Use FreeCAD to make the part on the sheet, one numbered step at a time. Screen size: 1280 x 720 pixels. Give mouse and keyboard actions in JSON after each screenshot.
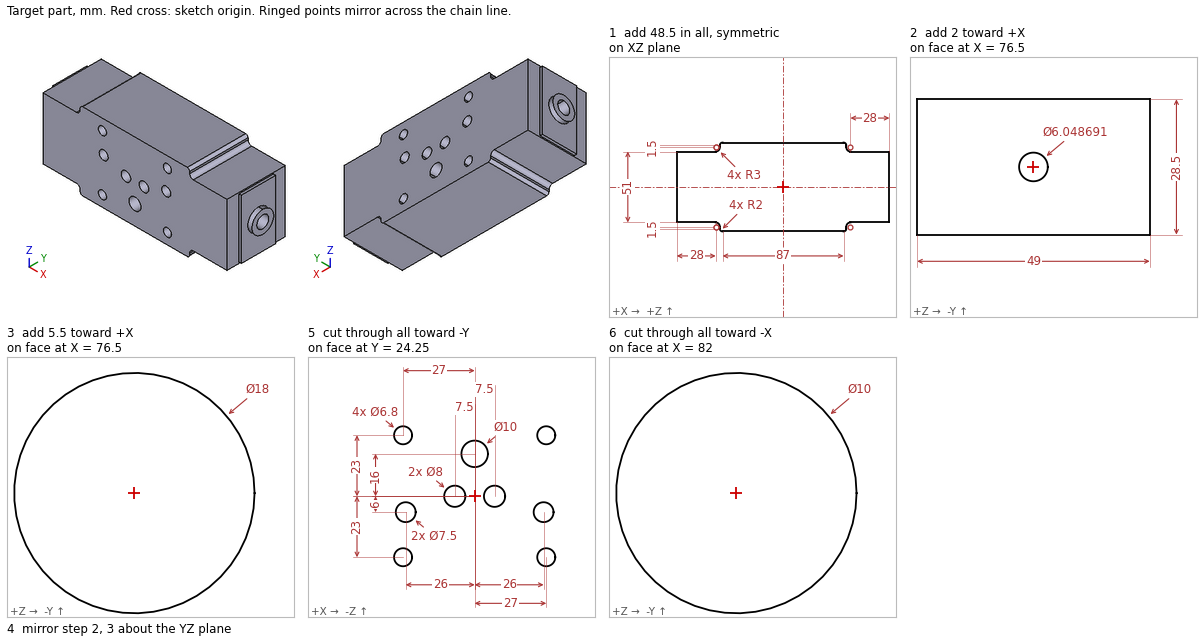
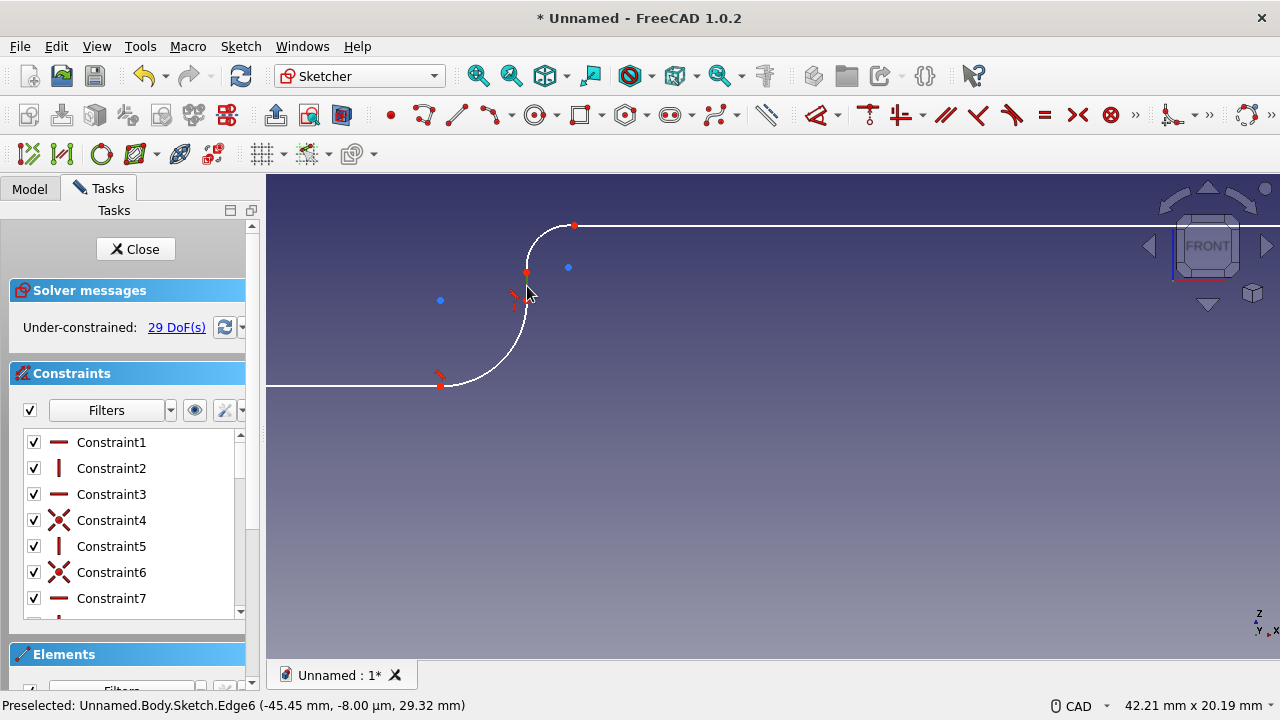
{"action": "left_click", "coordinate": [552, 229]}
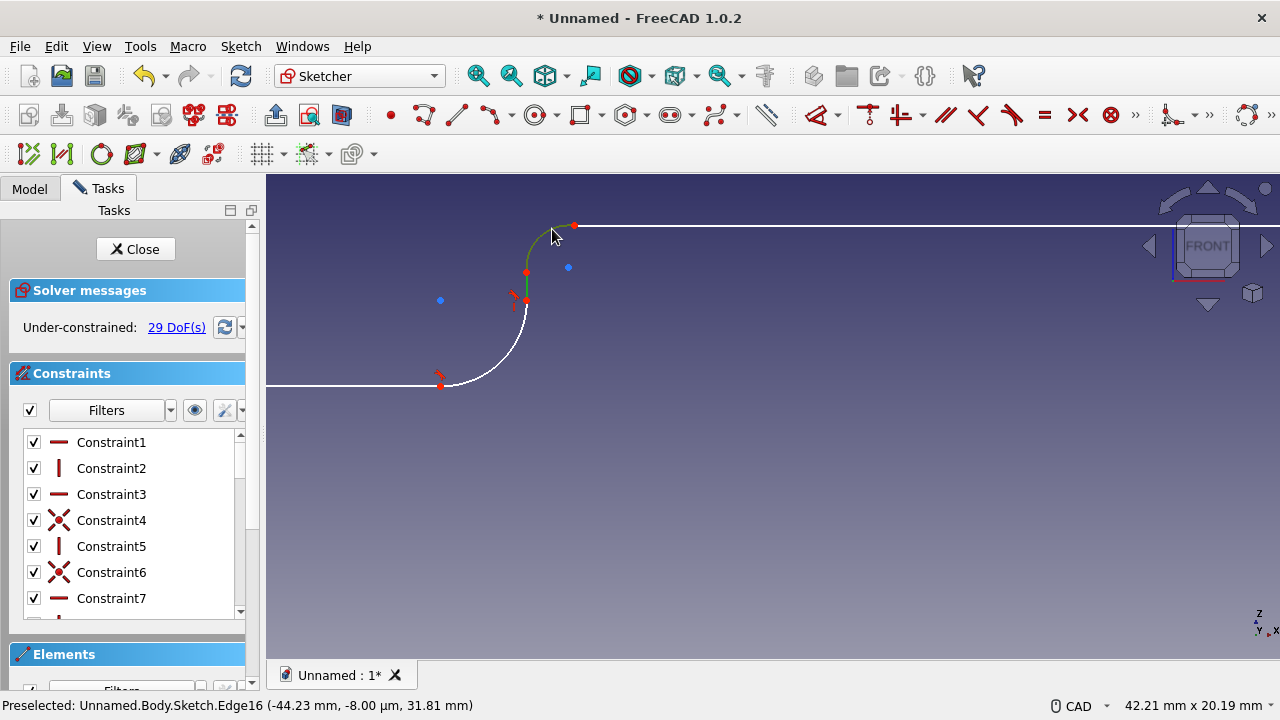
{"action": "left_click", "coordinate": [1012, 116]}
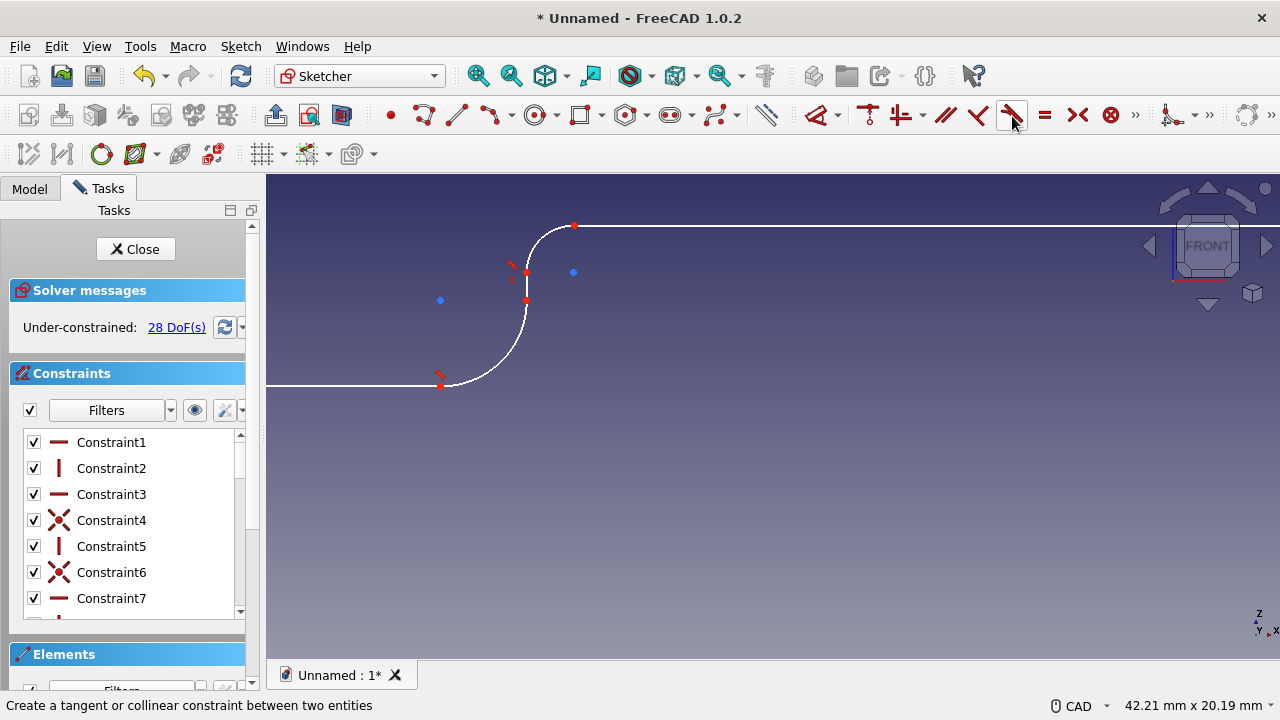
{"action": "scroll", "coordinate": [523, 303], "scroll_direction": "down", "scroll_amount": 9}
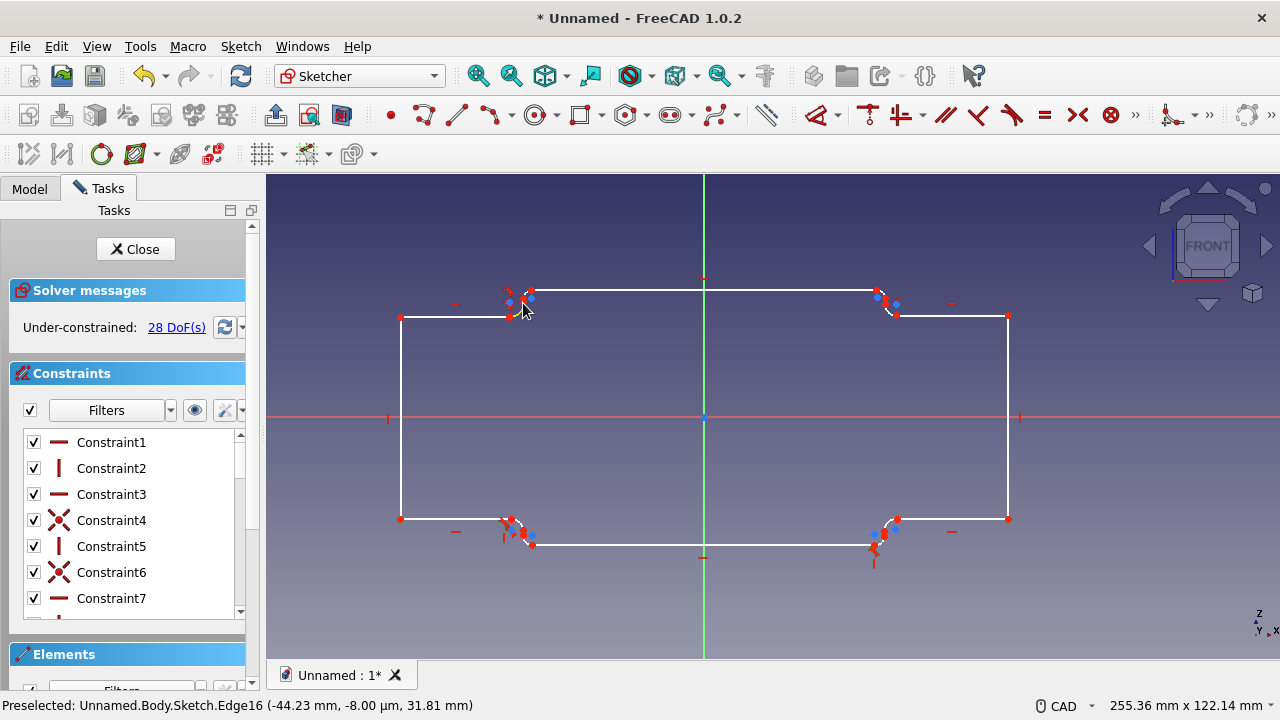
{"action": "left_click", "coordinate": [601, 290]}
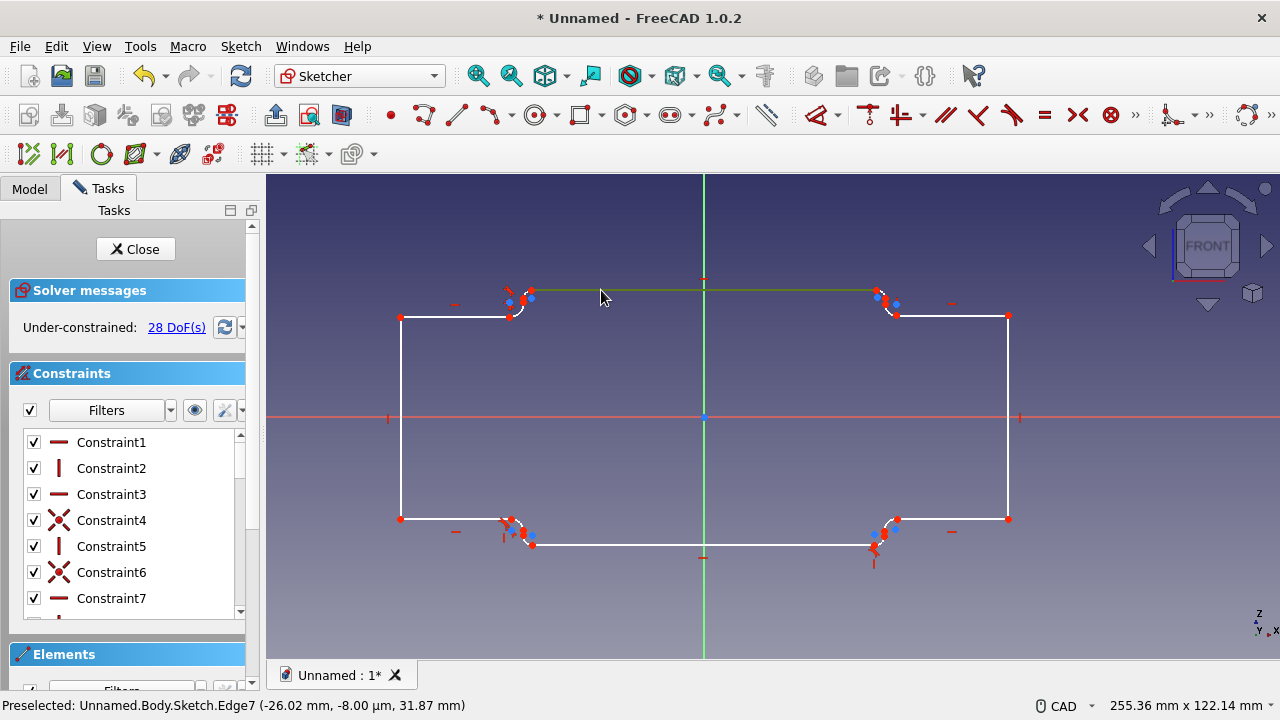
{"action": "scroll", "coordinate": [526, 293], "scroll_direction": "up", "scroll_amount": 5}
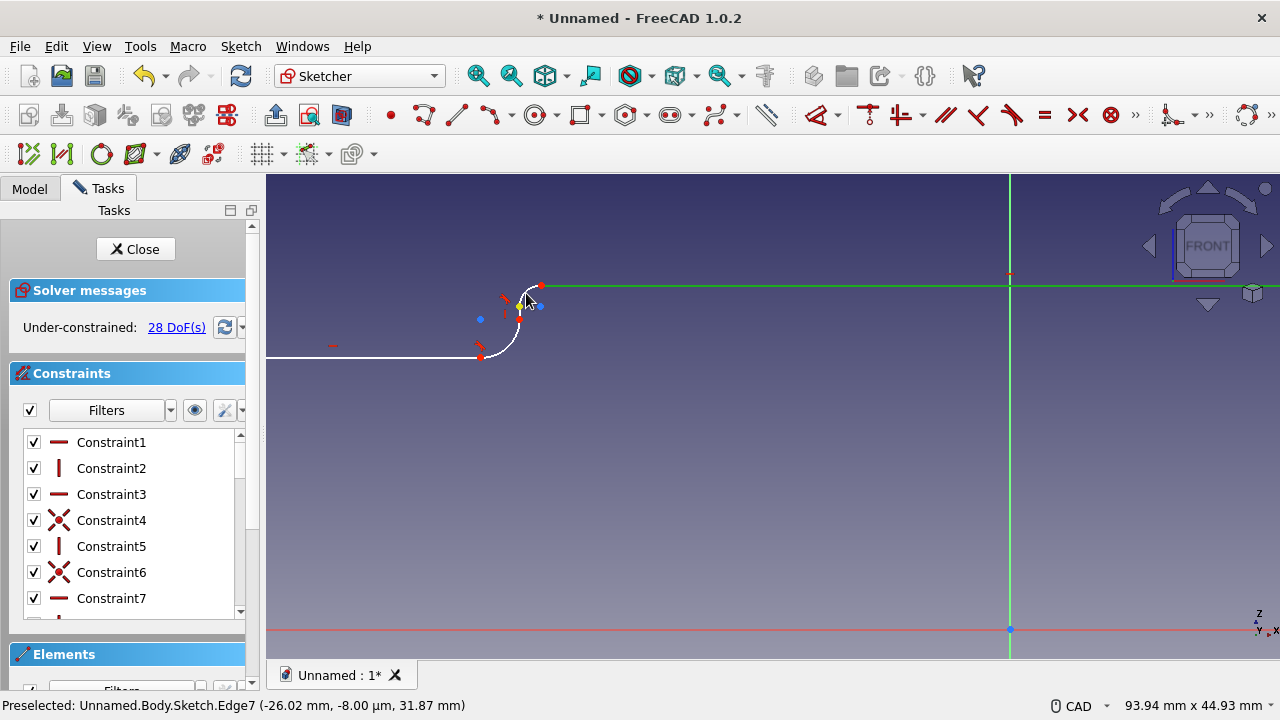
{"action": "left_click", "coordinate": [526, 292]}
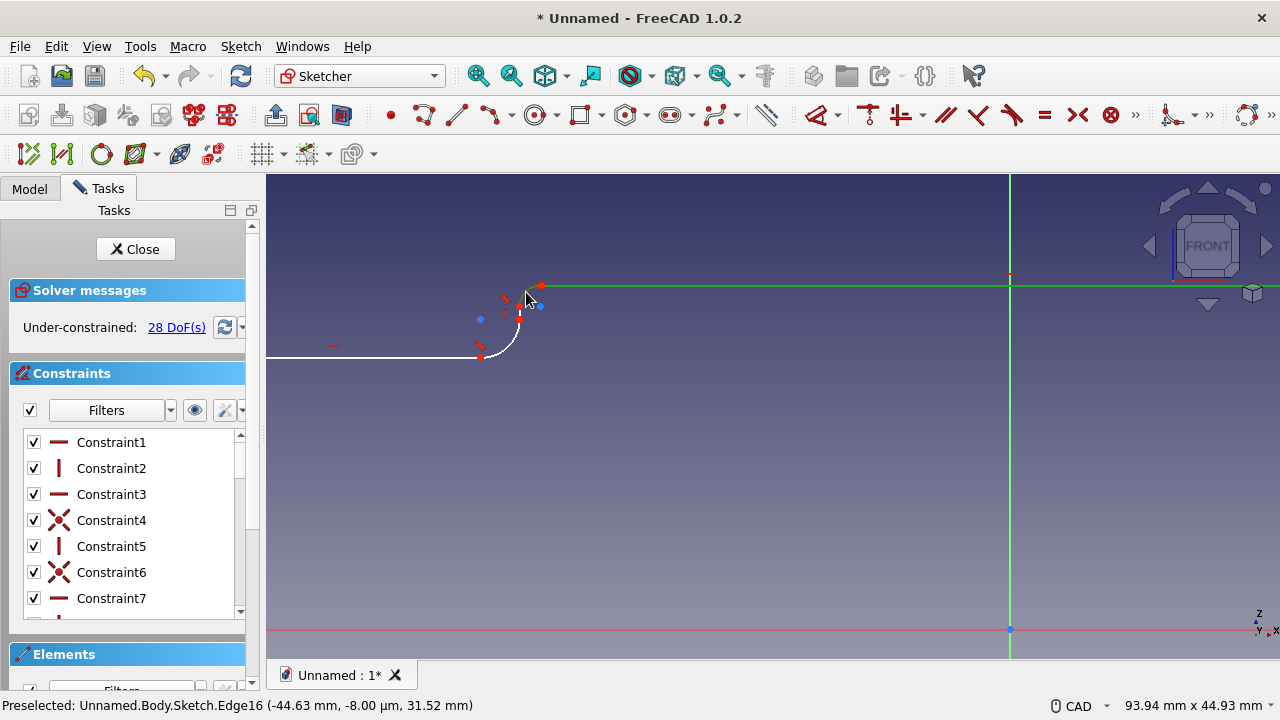
{"action": "left_click", "coordinate": [1012, 116]}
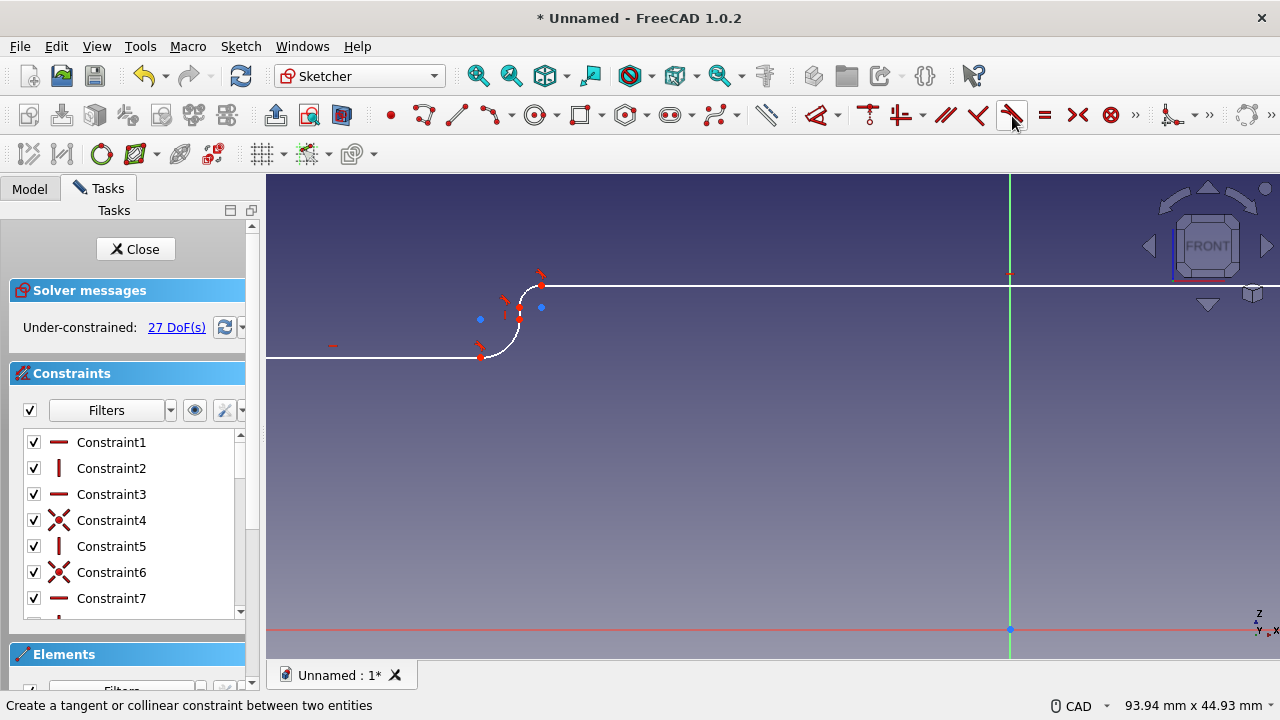
{"action": "left_click", "coordinate": [823, 286]}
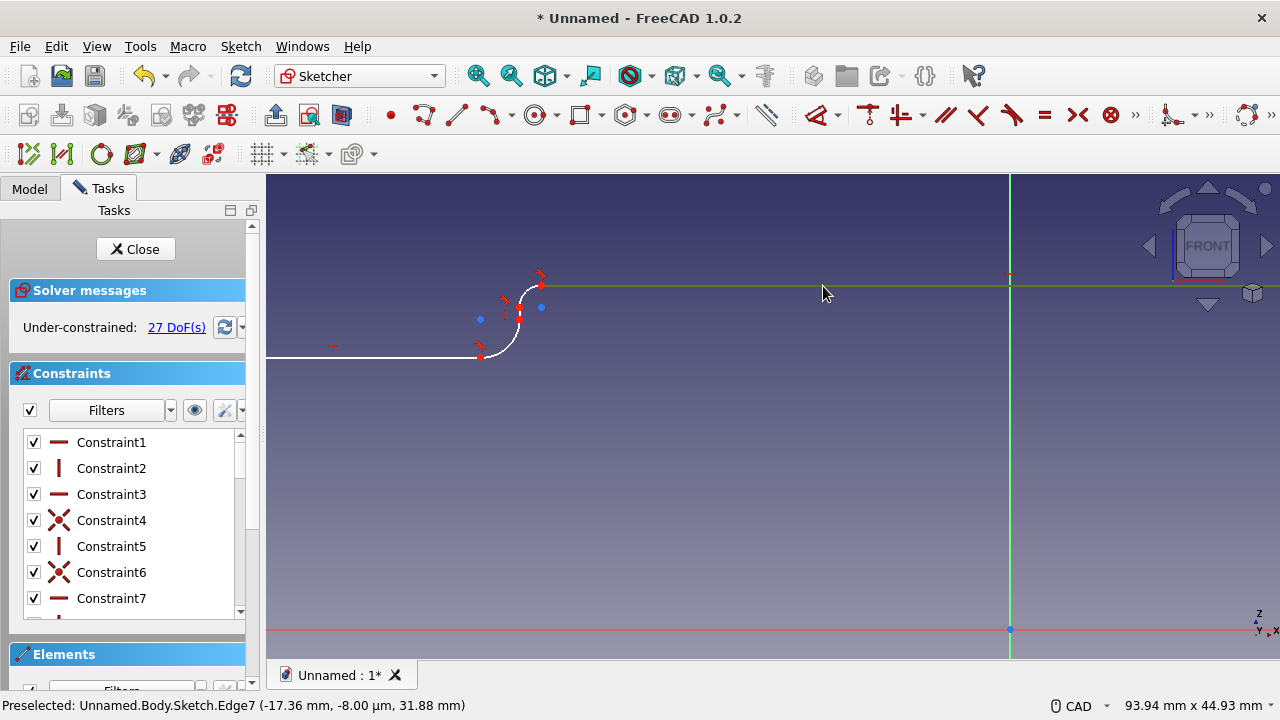
{"action": "scroll", "coordinate": [527, 292], "scroll_direction": "down", "scroll_amount": 5}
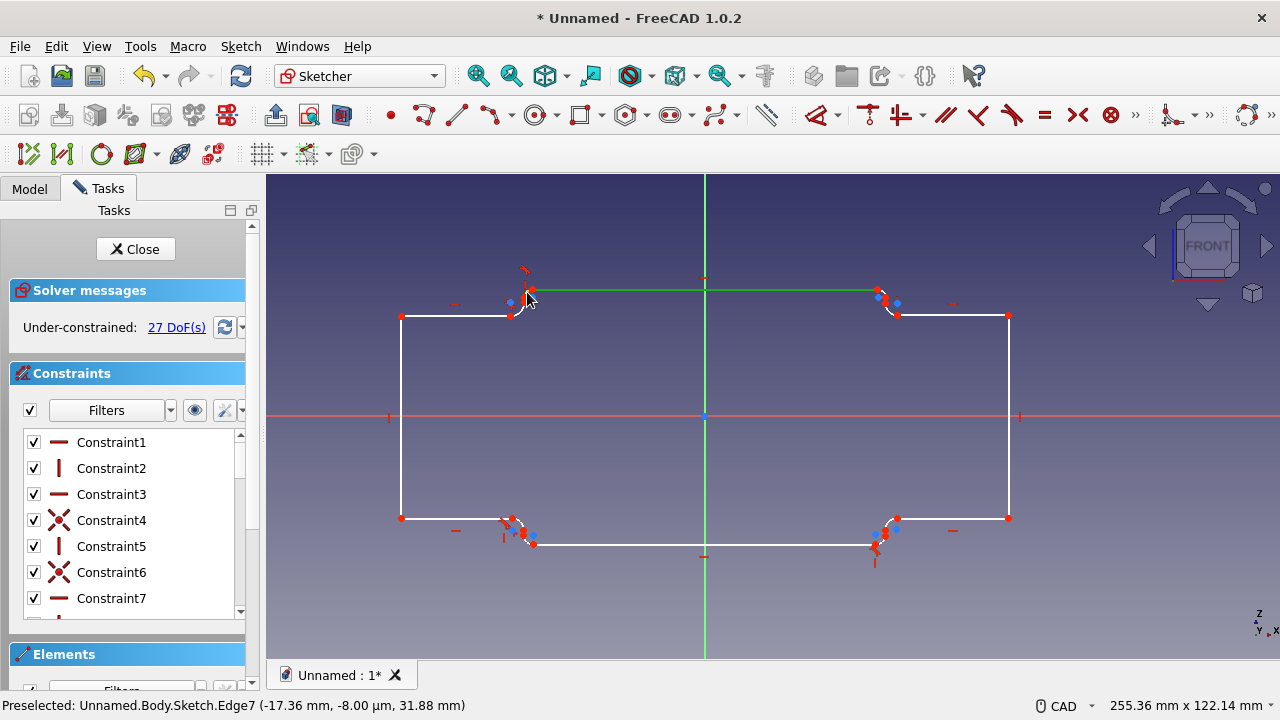
{"action": "scroll", "coordinate": [885, 294], "scroll_direction": "up", "scroll_amount": 7}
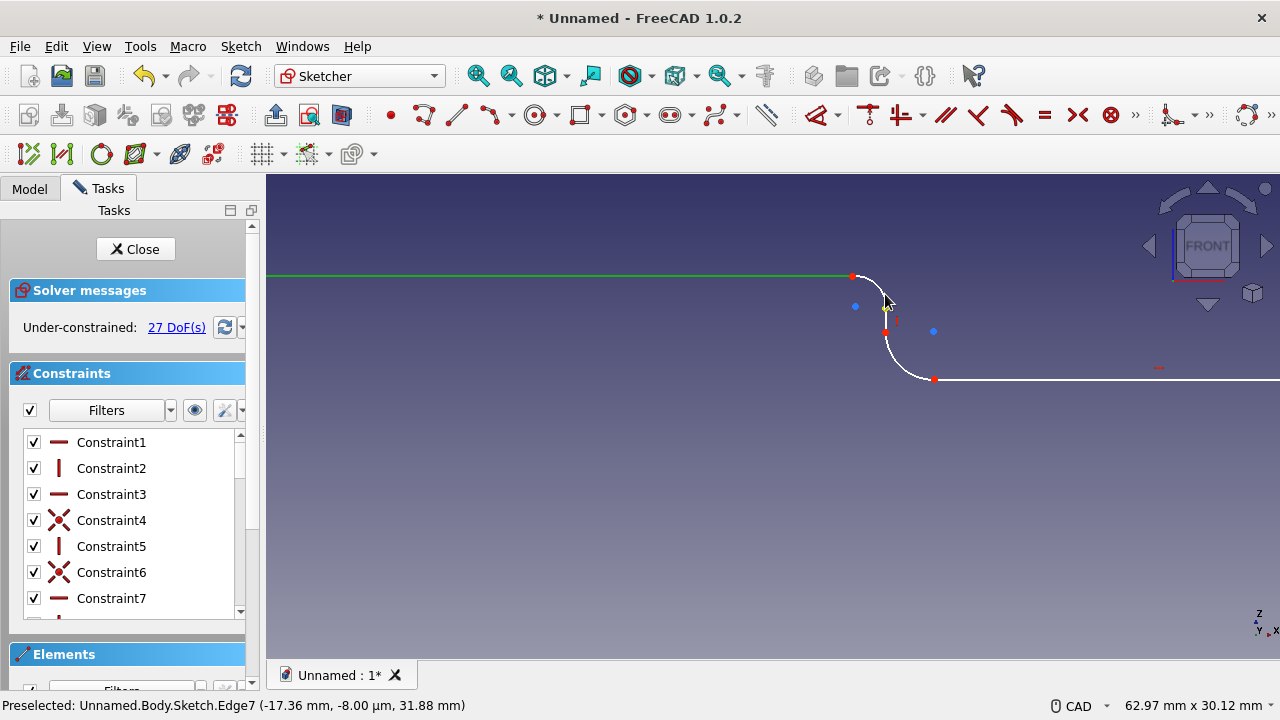
{"action": "left_click", "coordinate": [883, 293]}